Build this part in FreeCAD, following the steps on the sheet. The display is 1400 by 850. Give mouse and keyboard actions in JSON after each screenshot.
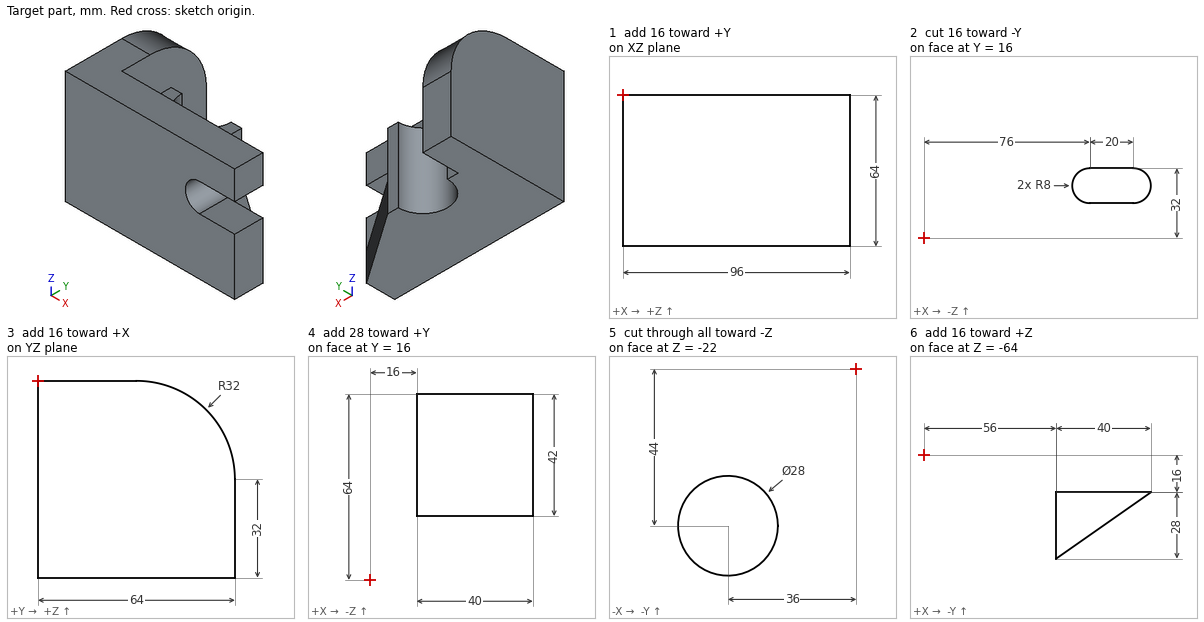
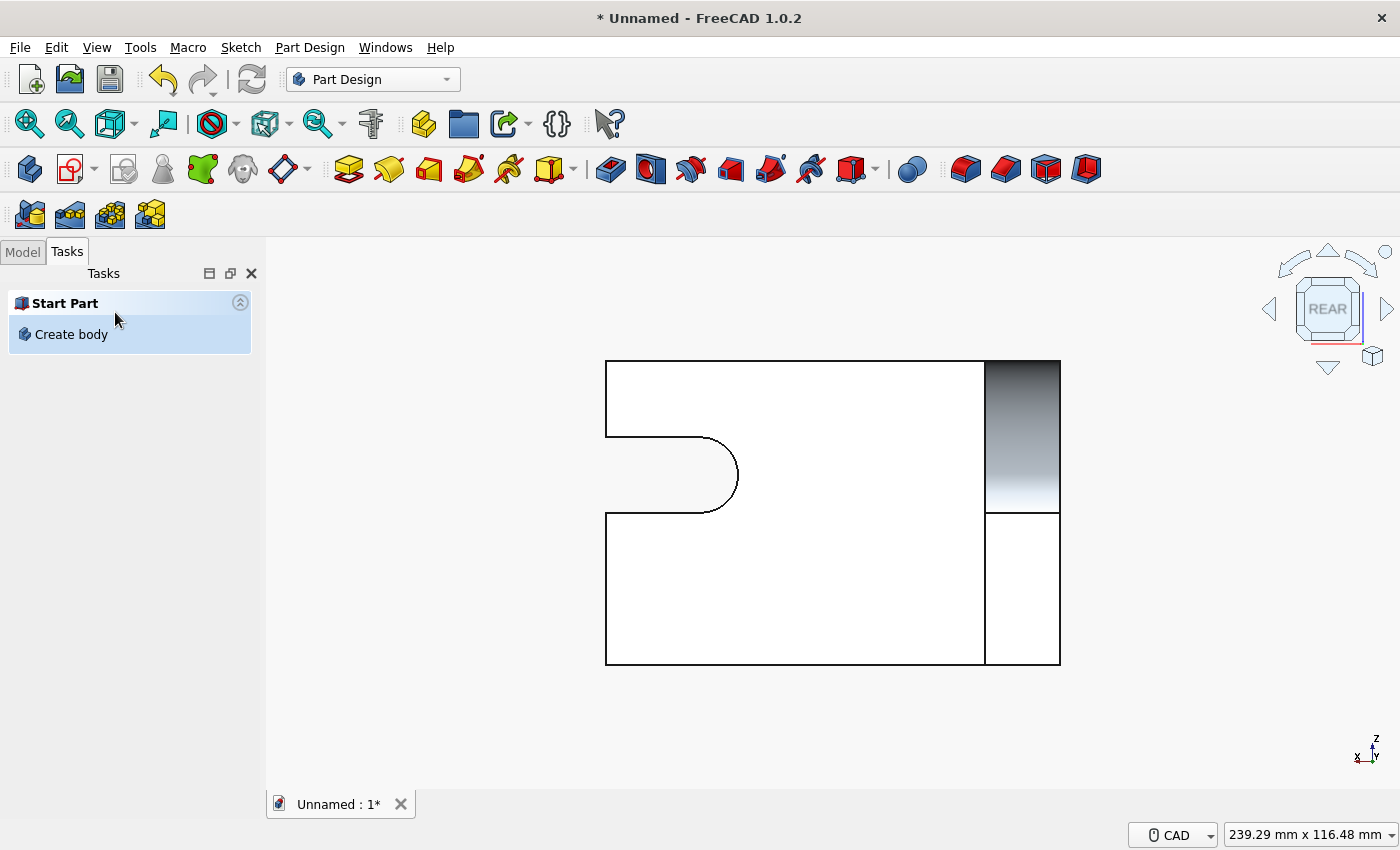
{"action": "left_click", "coordinate": [849, 512]}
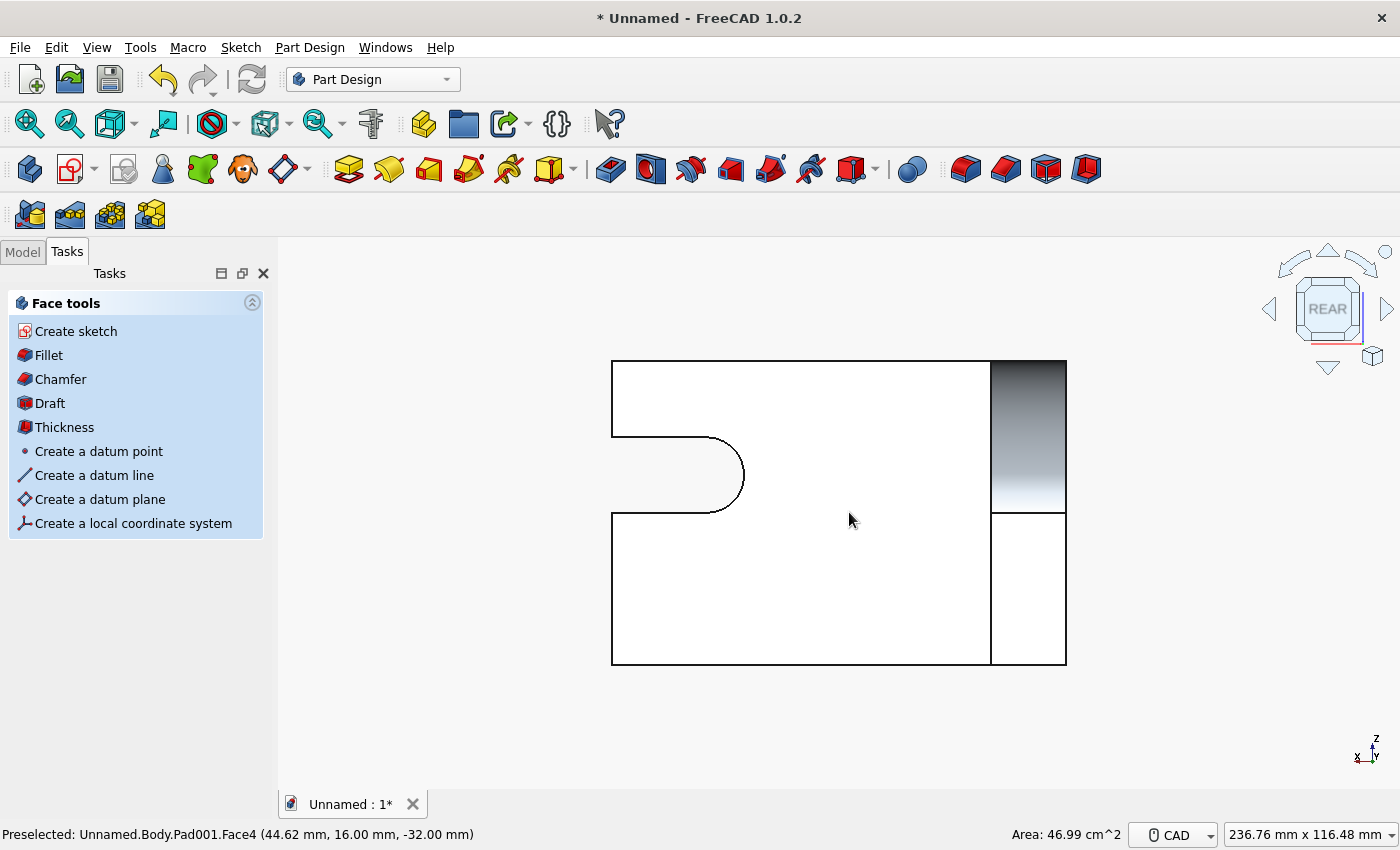
{"action": "left_click", "coordinate": [70, 170]}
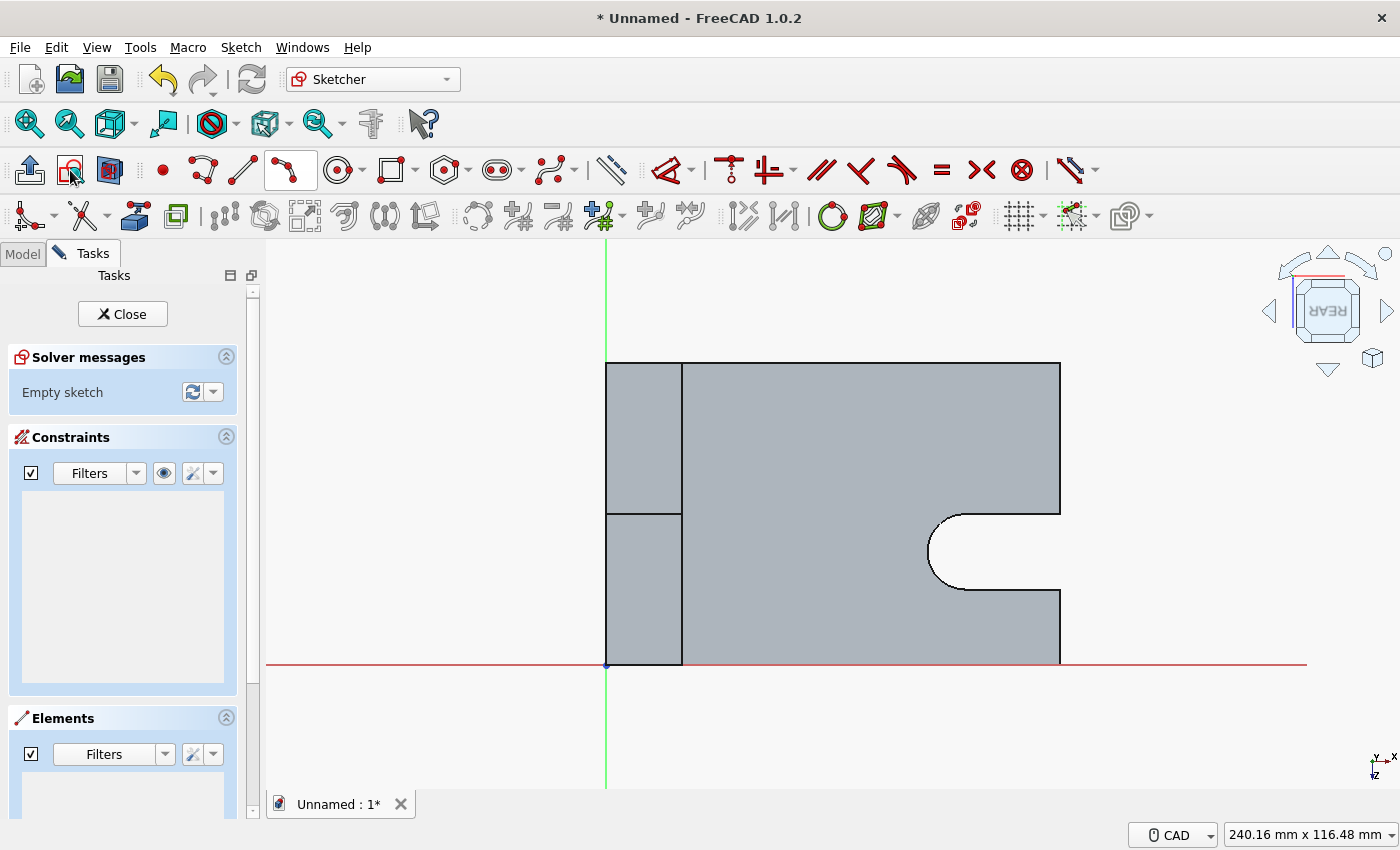
{"action": "key", "text": "q s"}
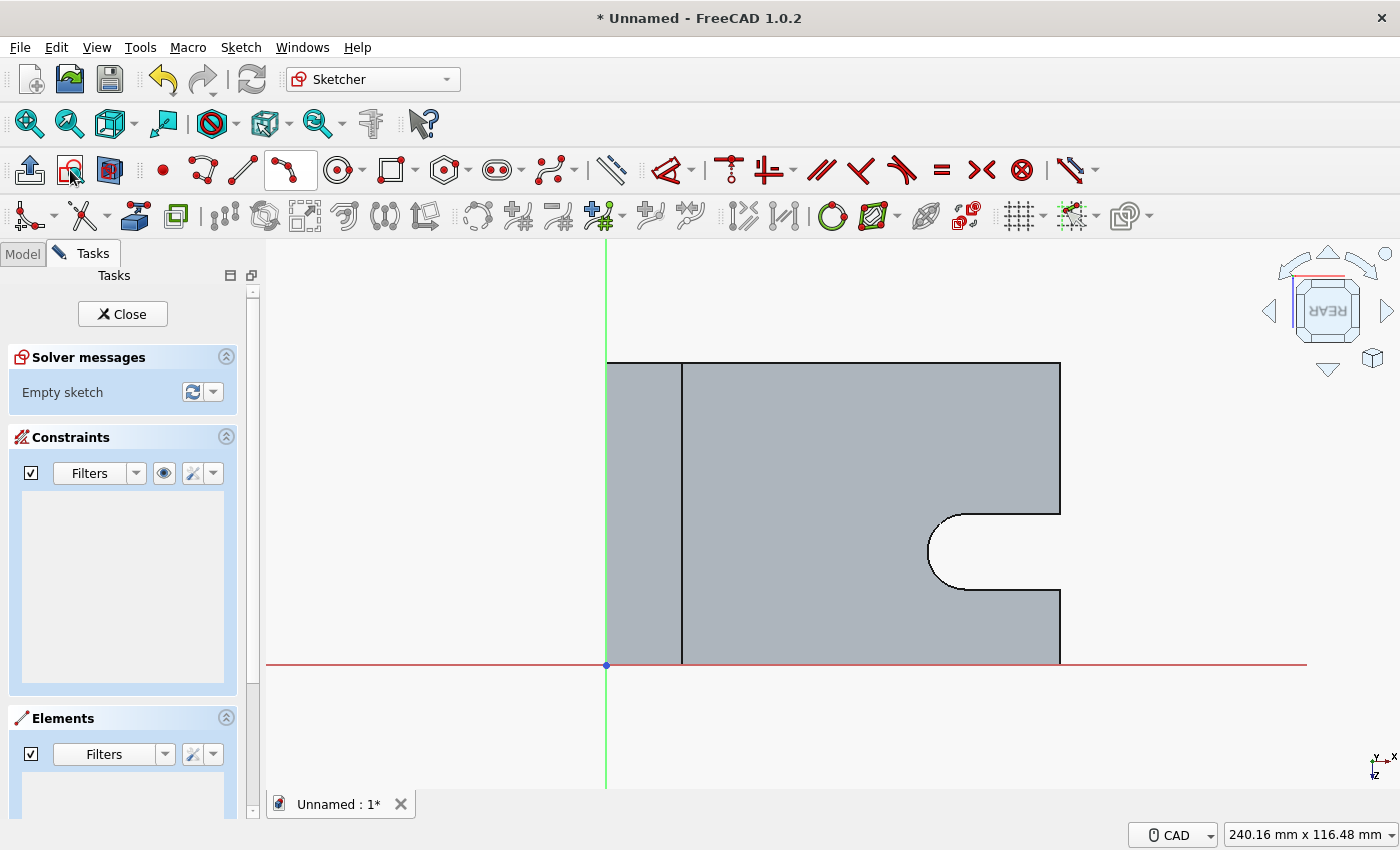
{"action": "left_click", "coordinate": [392, 170]}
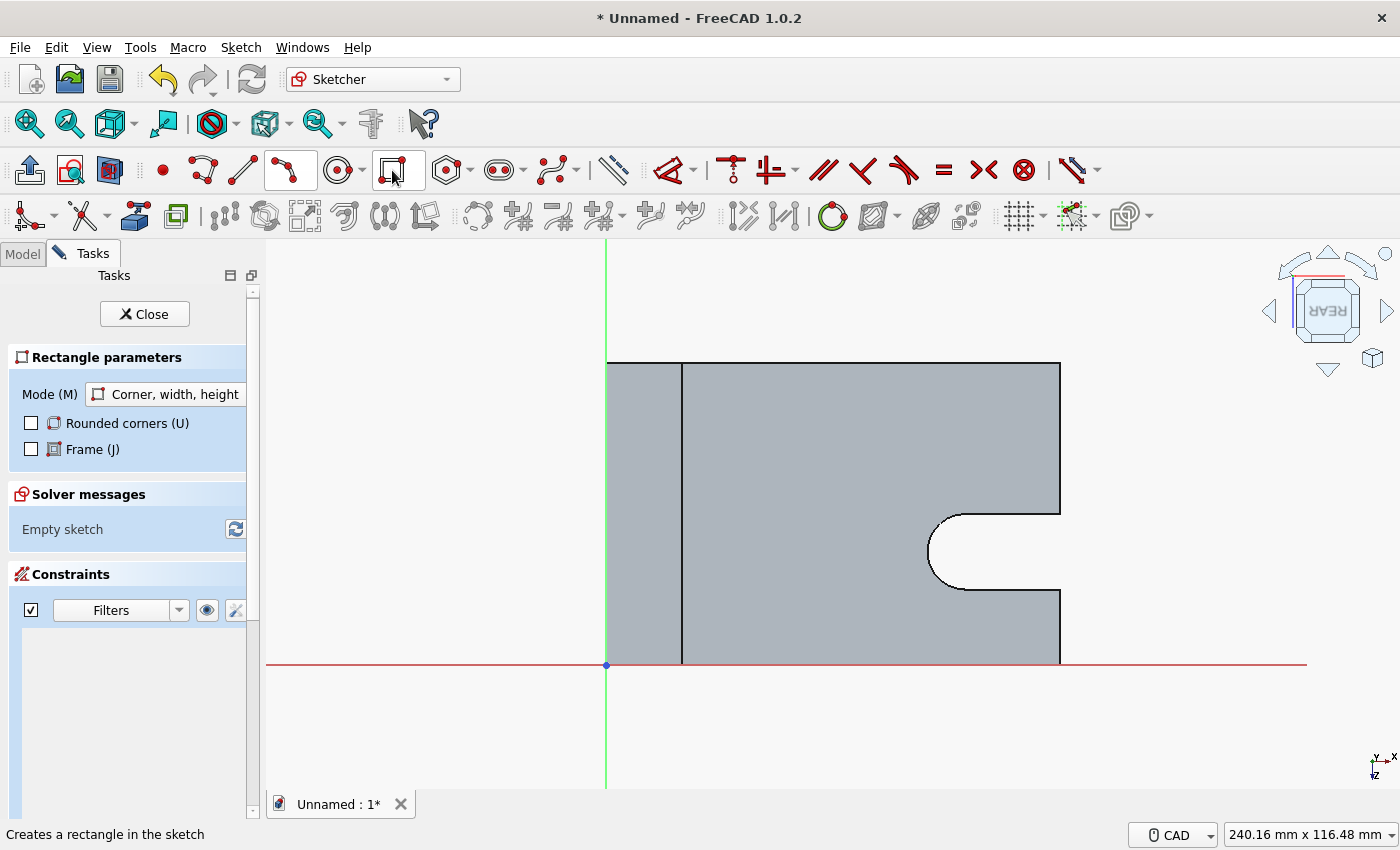
{"action": "left_click", "coordinate": [682, 363]}
{"action": "mouse_move", "coordinate": [871, 561]}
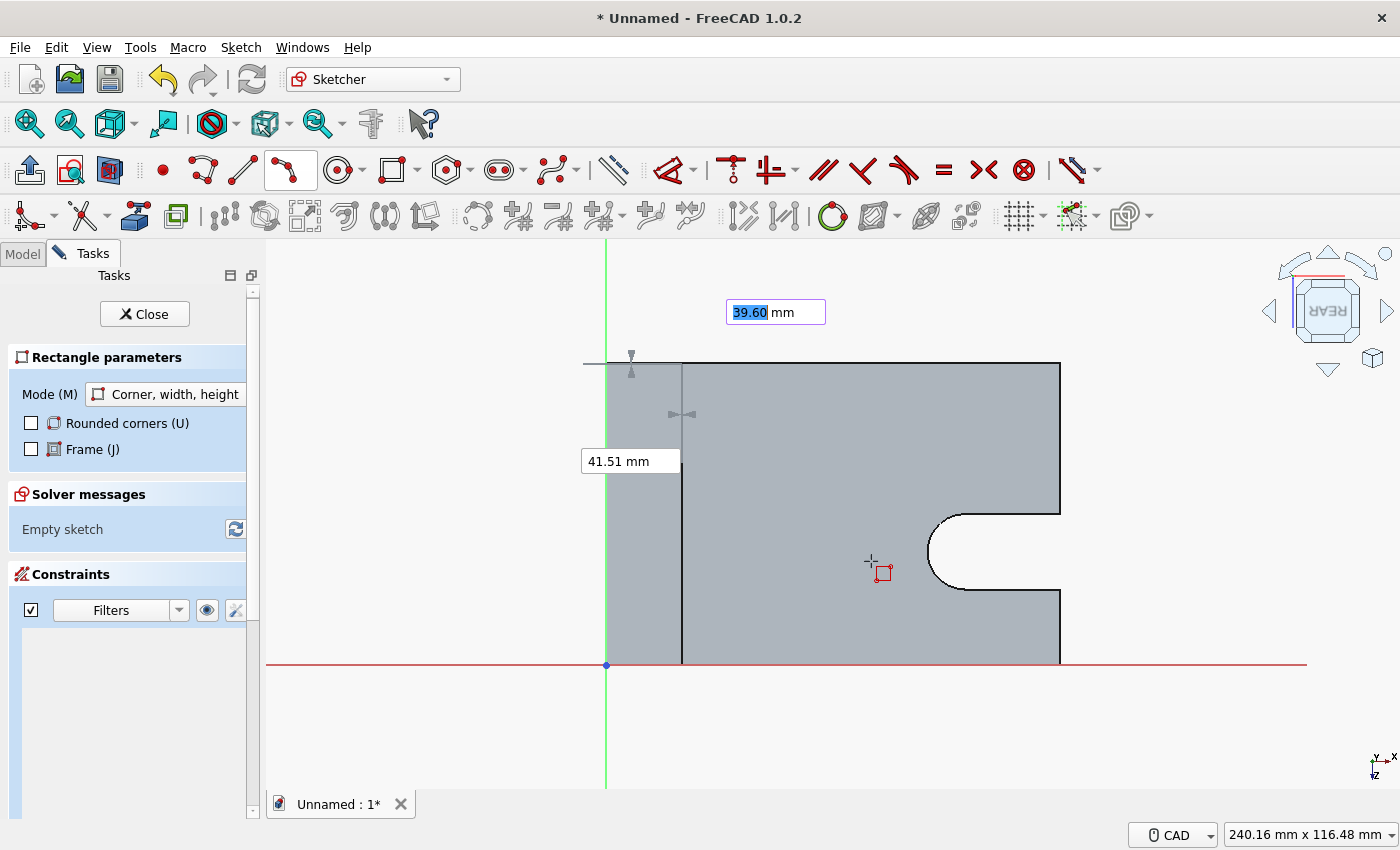
{"action": "type", "text": "40"}
{"action": "key", "text": "Tab"}
{"action": "type", "text": "42"}
{"action": "key", "text": "Return"}
{"action": "key", "text": "Escape"}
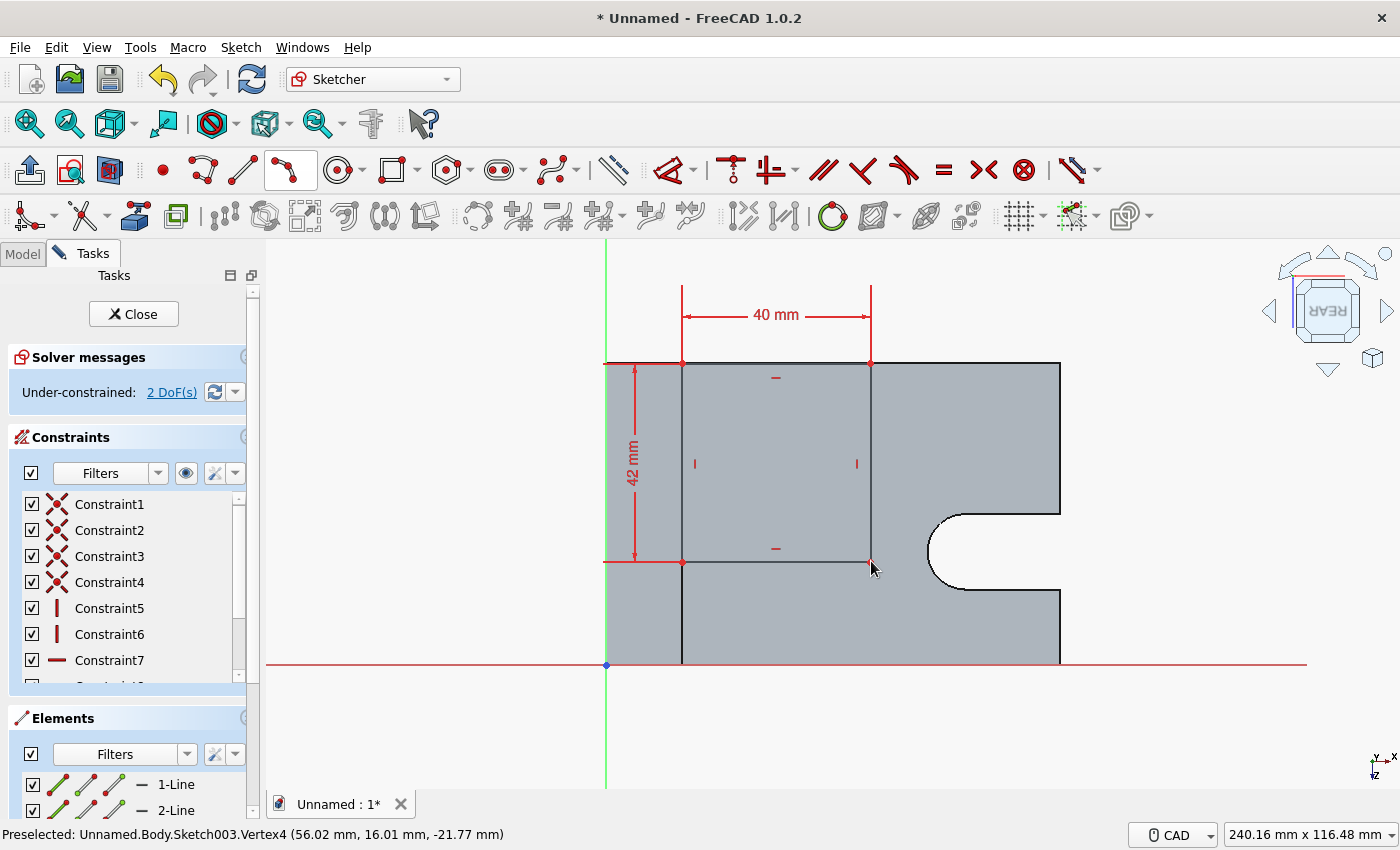
{"action": "left_click", "coordinate": [668, 170]}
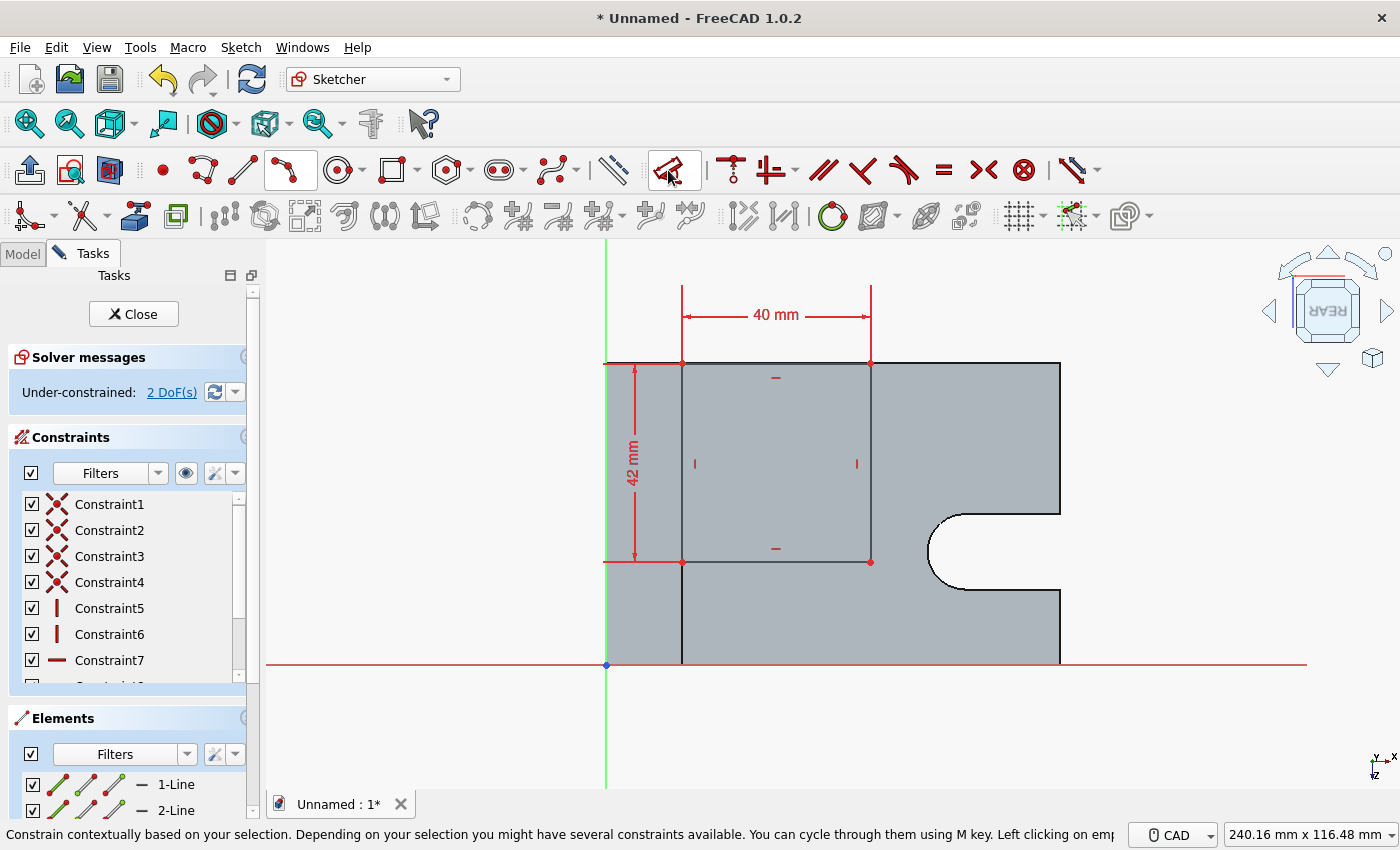
{"action": "left_click", "coordinate": [682, 364]}
{"action": "left_click", "coordinate": [644, 699]}